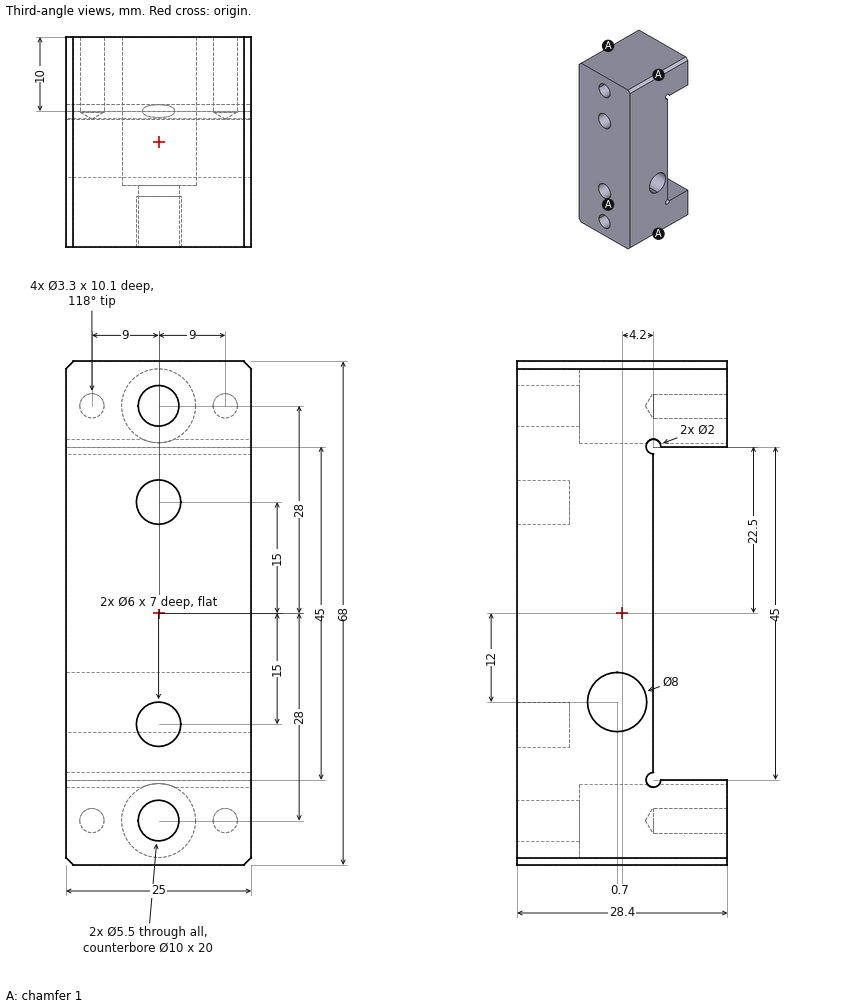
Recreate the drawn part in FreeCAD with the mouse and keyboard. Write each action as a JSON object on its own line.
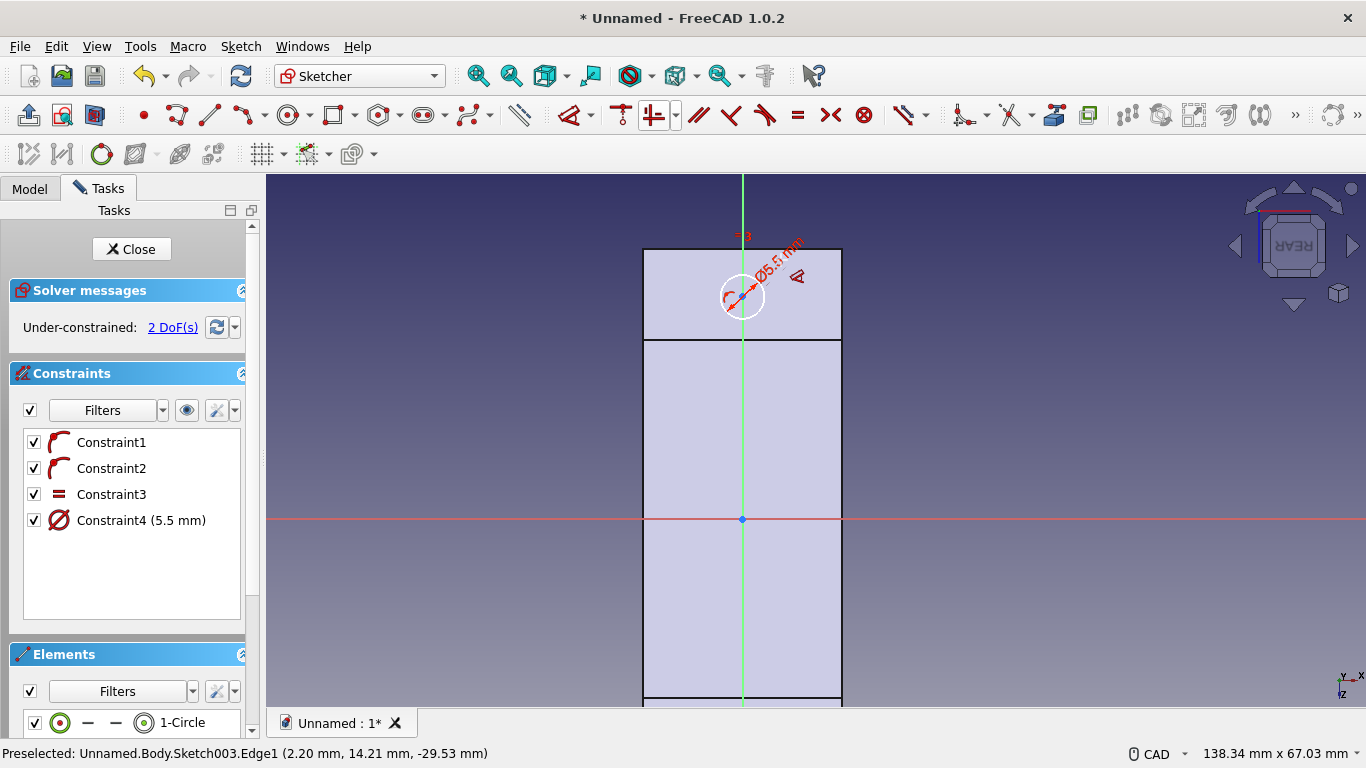
{"action": "left_click", "coordinate": [743, 297]}
{"action": "left_click", "coordinate": [777, 408]}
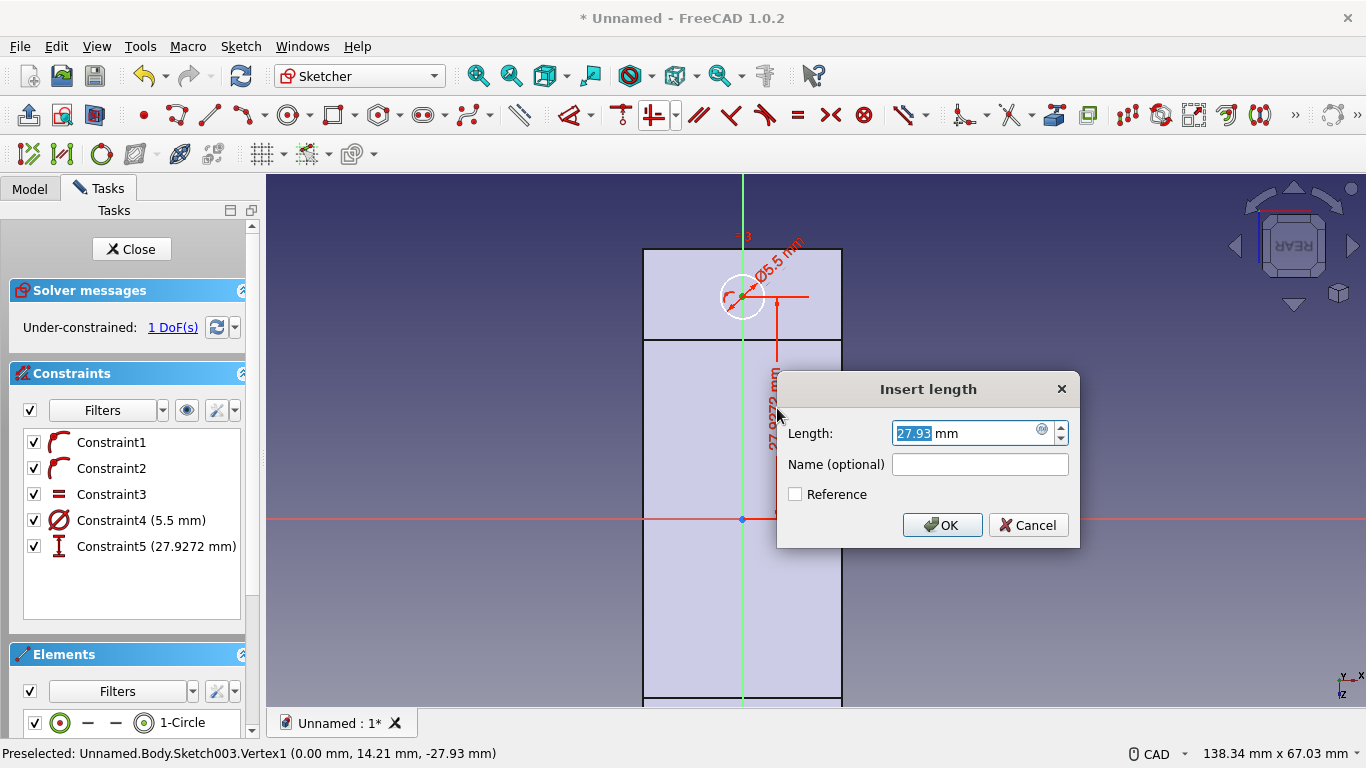
{"action": "type", "text": "28"}
{"action": "key", "text": "Return"}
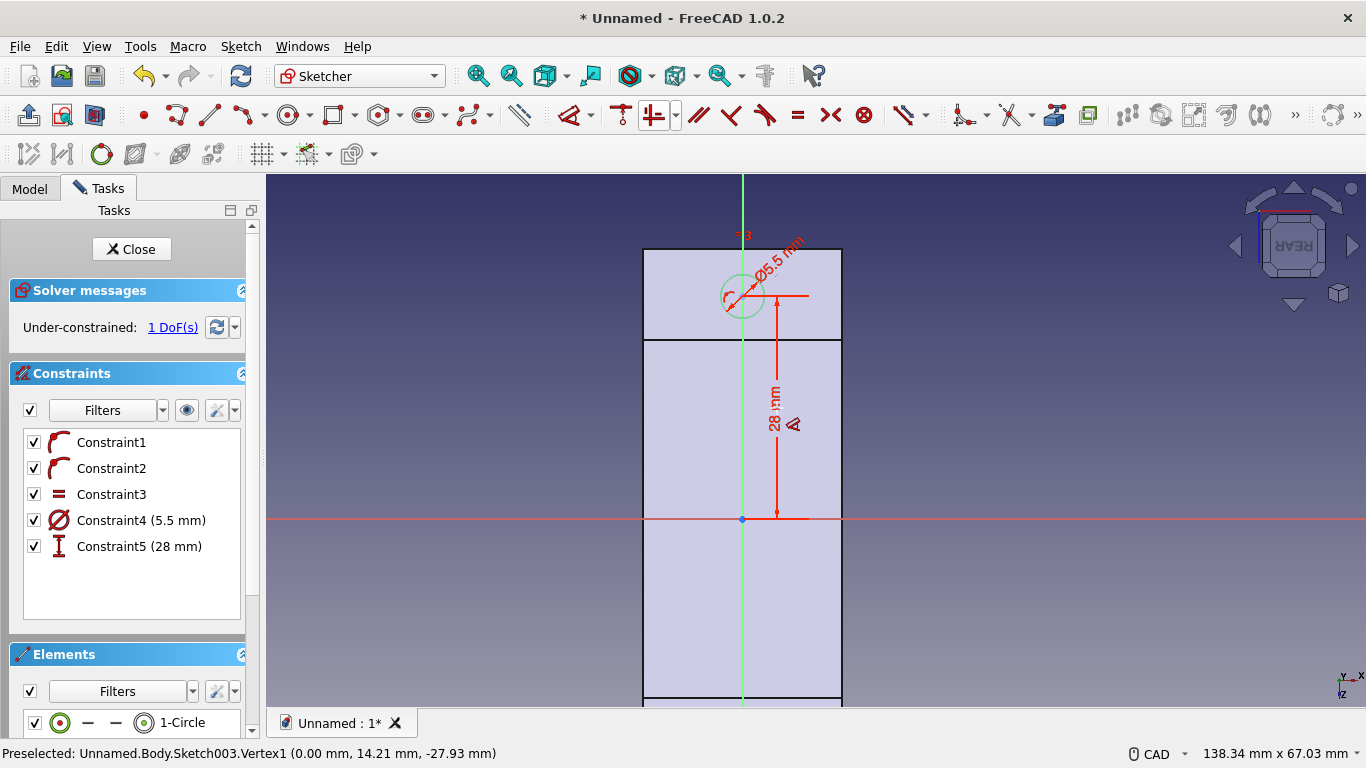
{"action": "scroll", "coordinate": [758, 281], "scroll_direction": "down", "scroll_amount": 2}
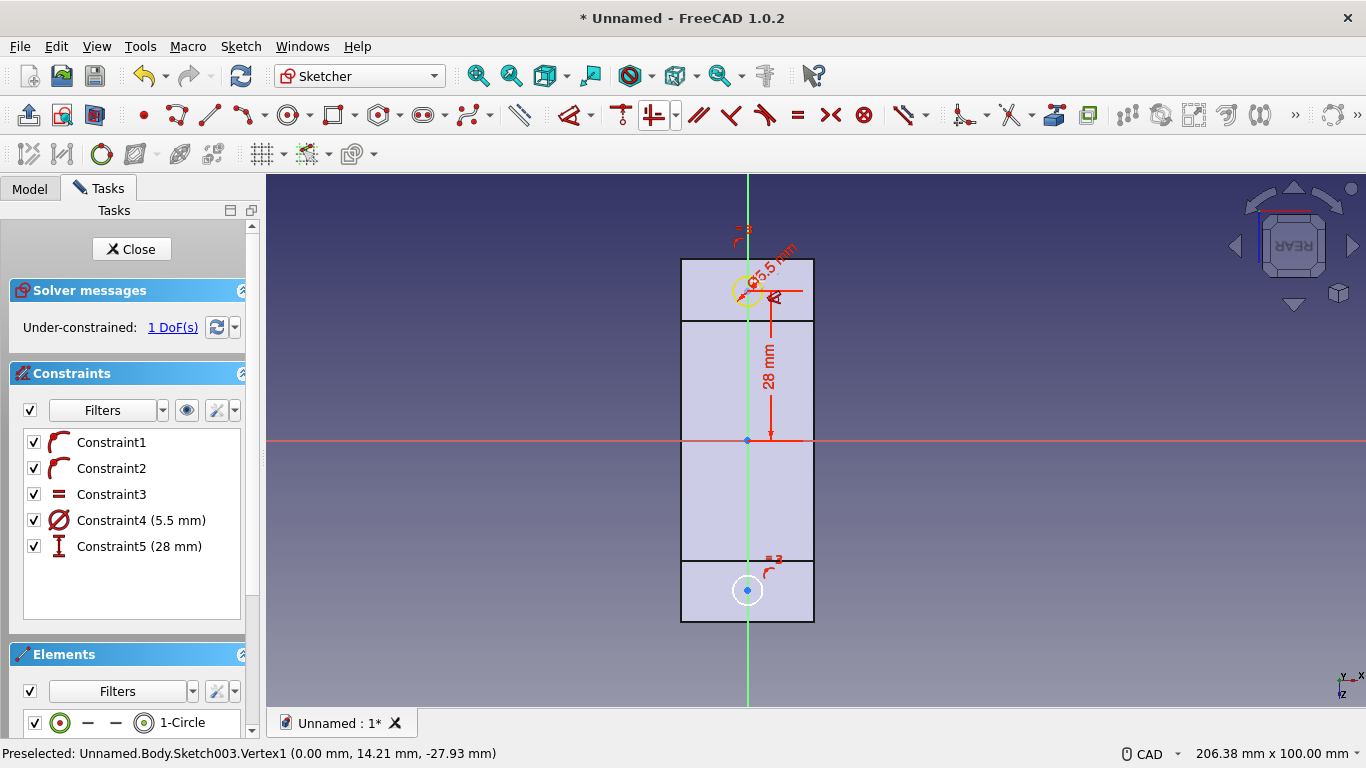
{"action": "left_click", "coordinate": [748, 590]}
{"action": "left_click", "coordinate": [782, 516]}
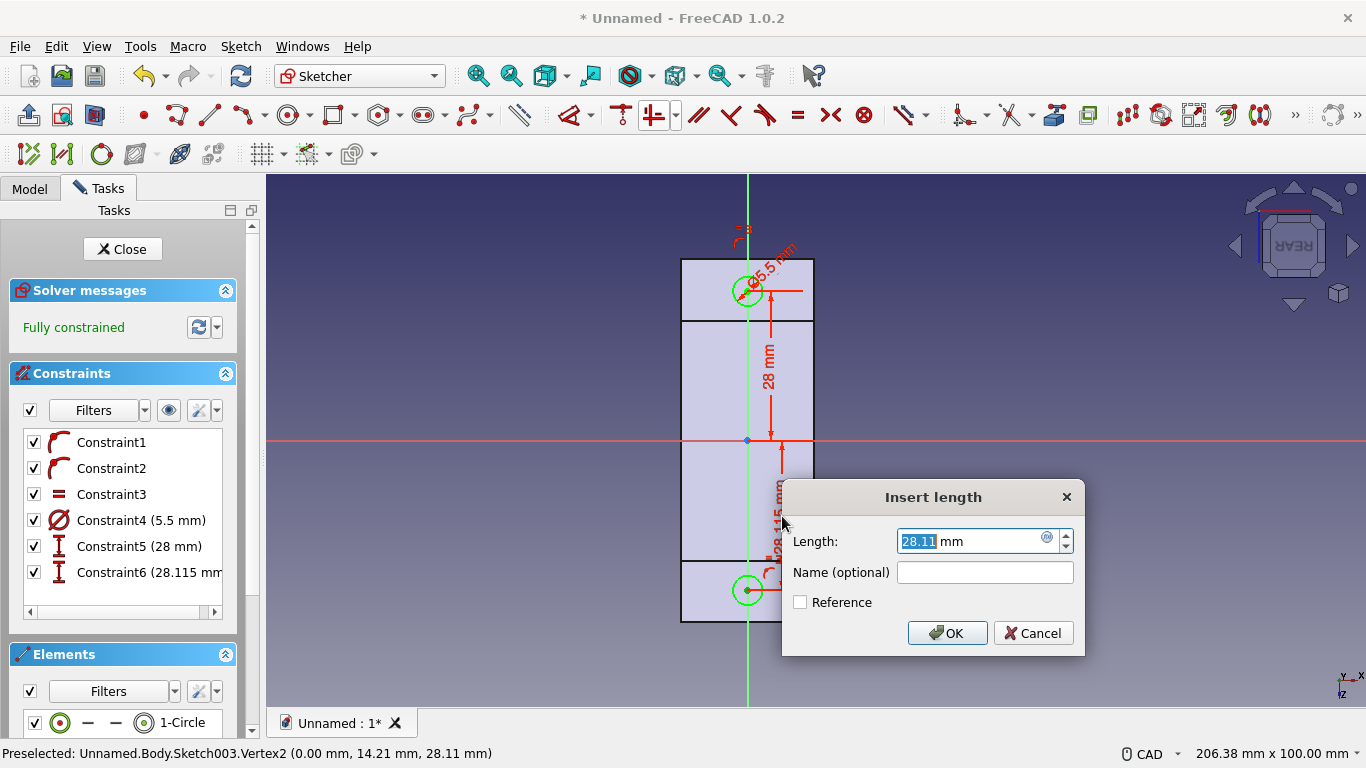
{"action": "type", "text": "28"}
{"action": "key", "text": "Return"}
{"action": "key", "text": "Escape"}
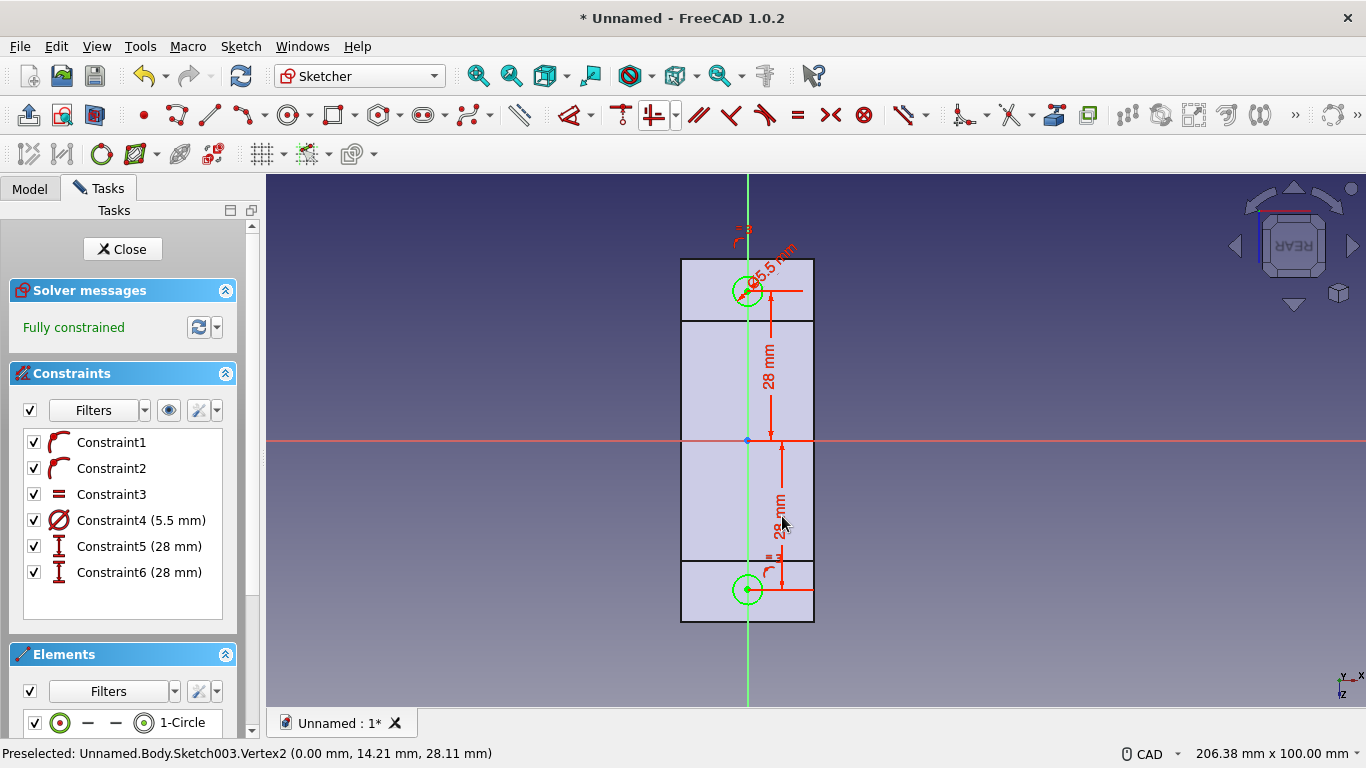
{"action": "left_click", "coordinate": [123, 249]}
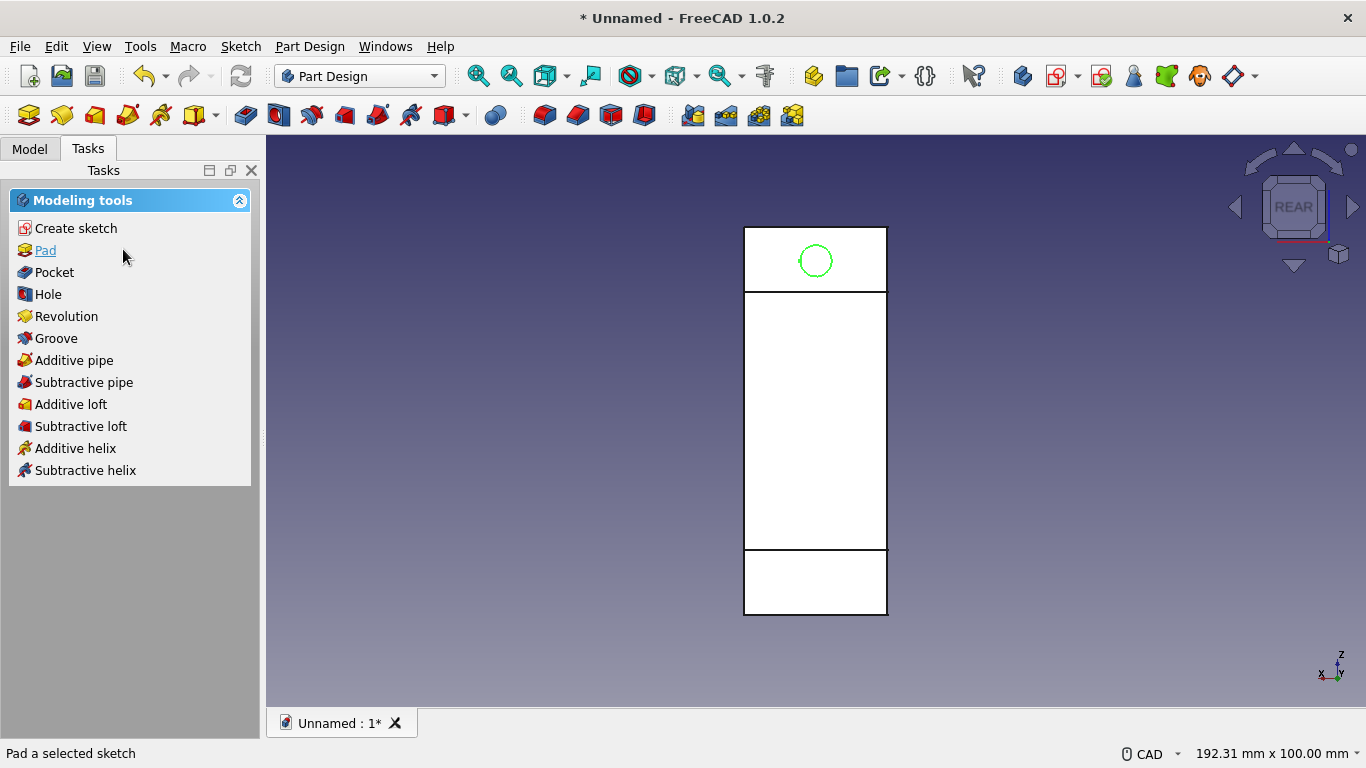
{"action": "left_click", "coordinate": [279, 116]}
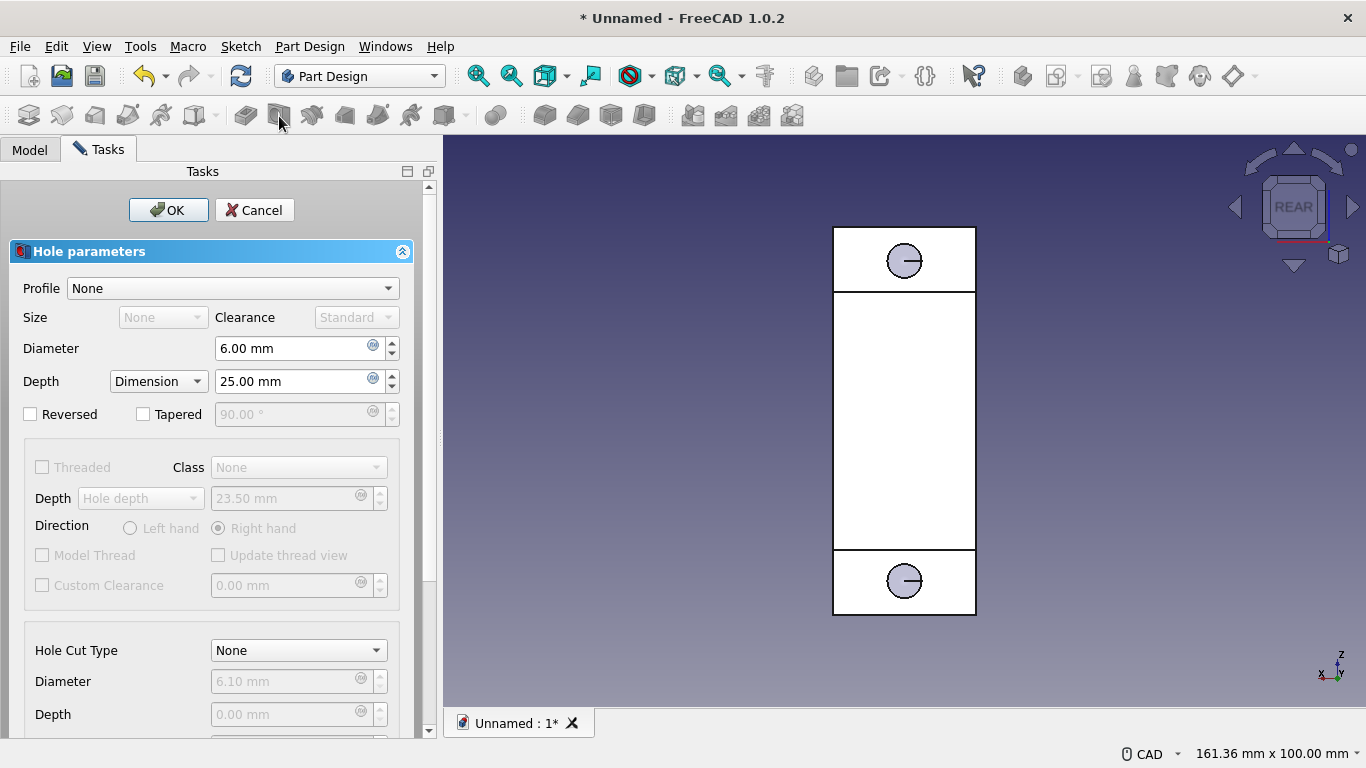
{"action": "triple_click", "coordinate": [300, 348]}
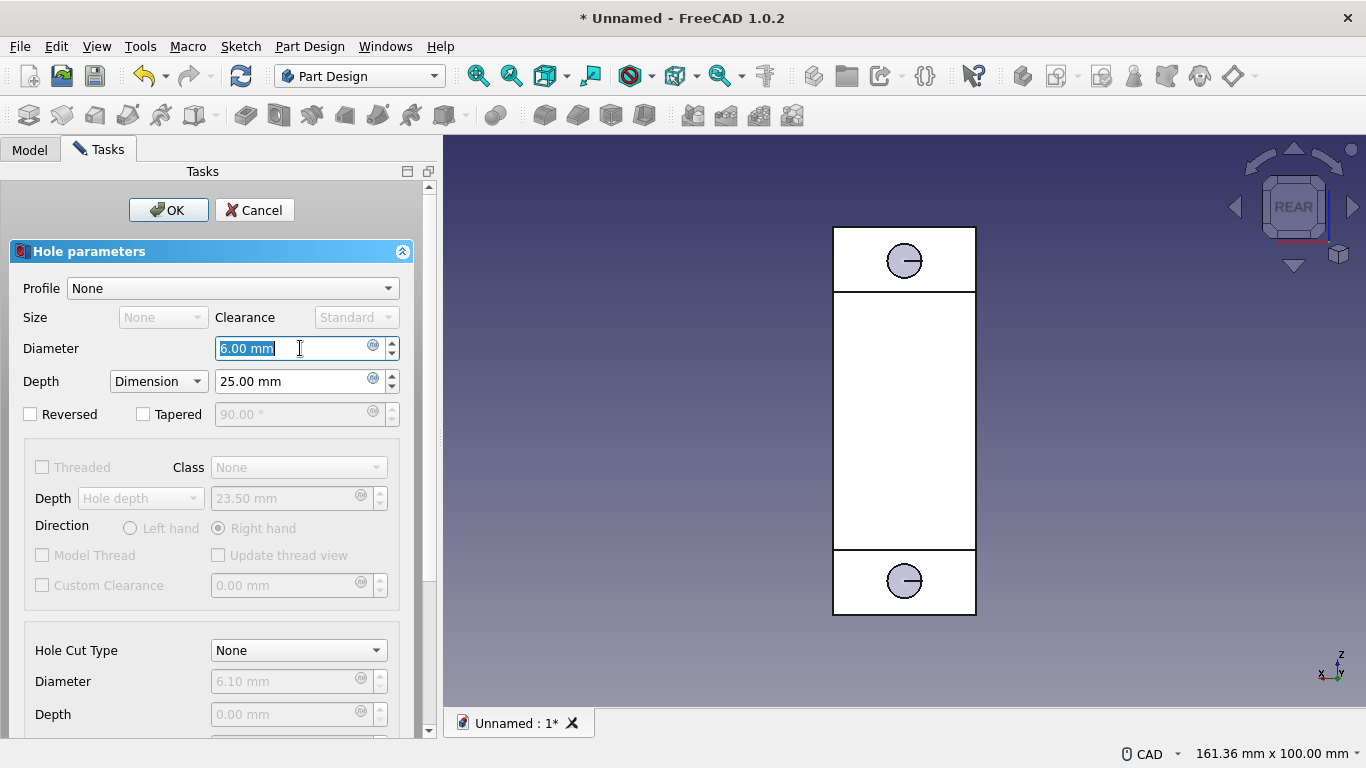
{"action": "type", "text": "5.5"}
{"action": "key", "text": "Tab"}